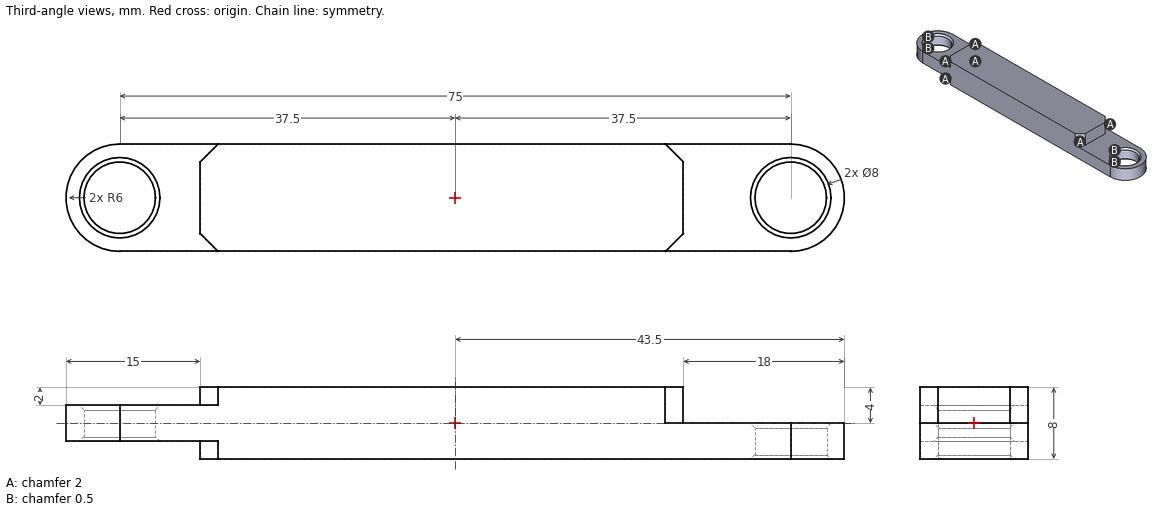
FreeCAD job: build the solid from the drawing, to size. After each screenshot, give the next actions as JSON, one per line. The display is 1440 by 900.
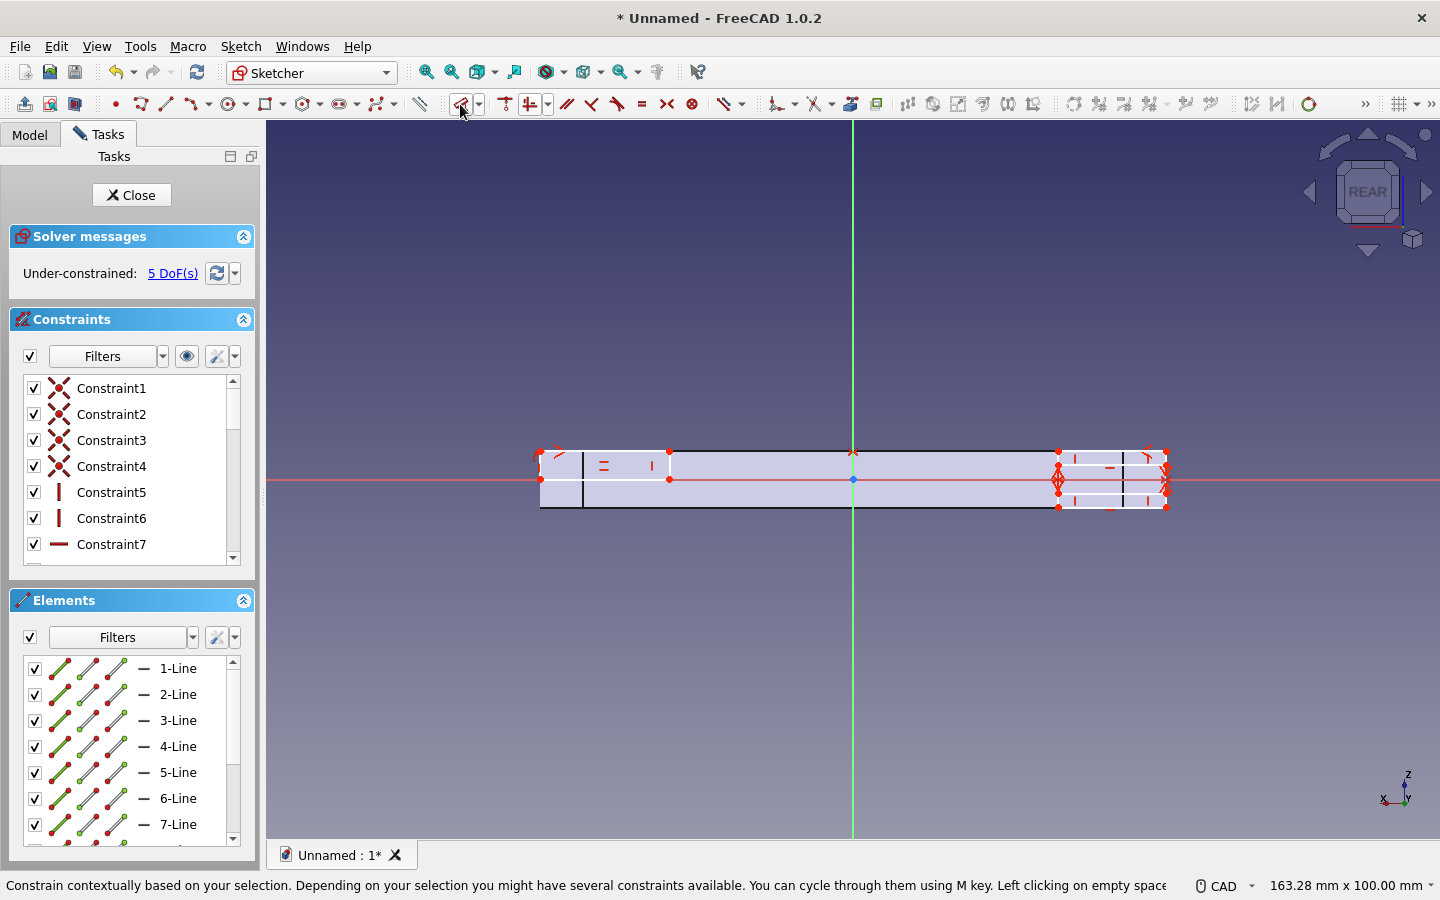
{"action": "scroll", "coordinate": [540, 463], "scroll_direction": "up", "scroll_amount": 2}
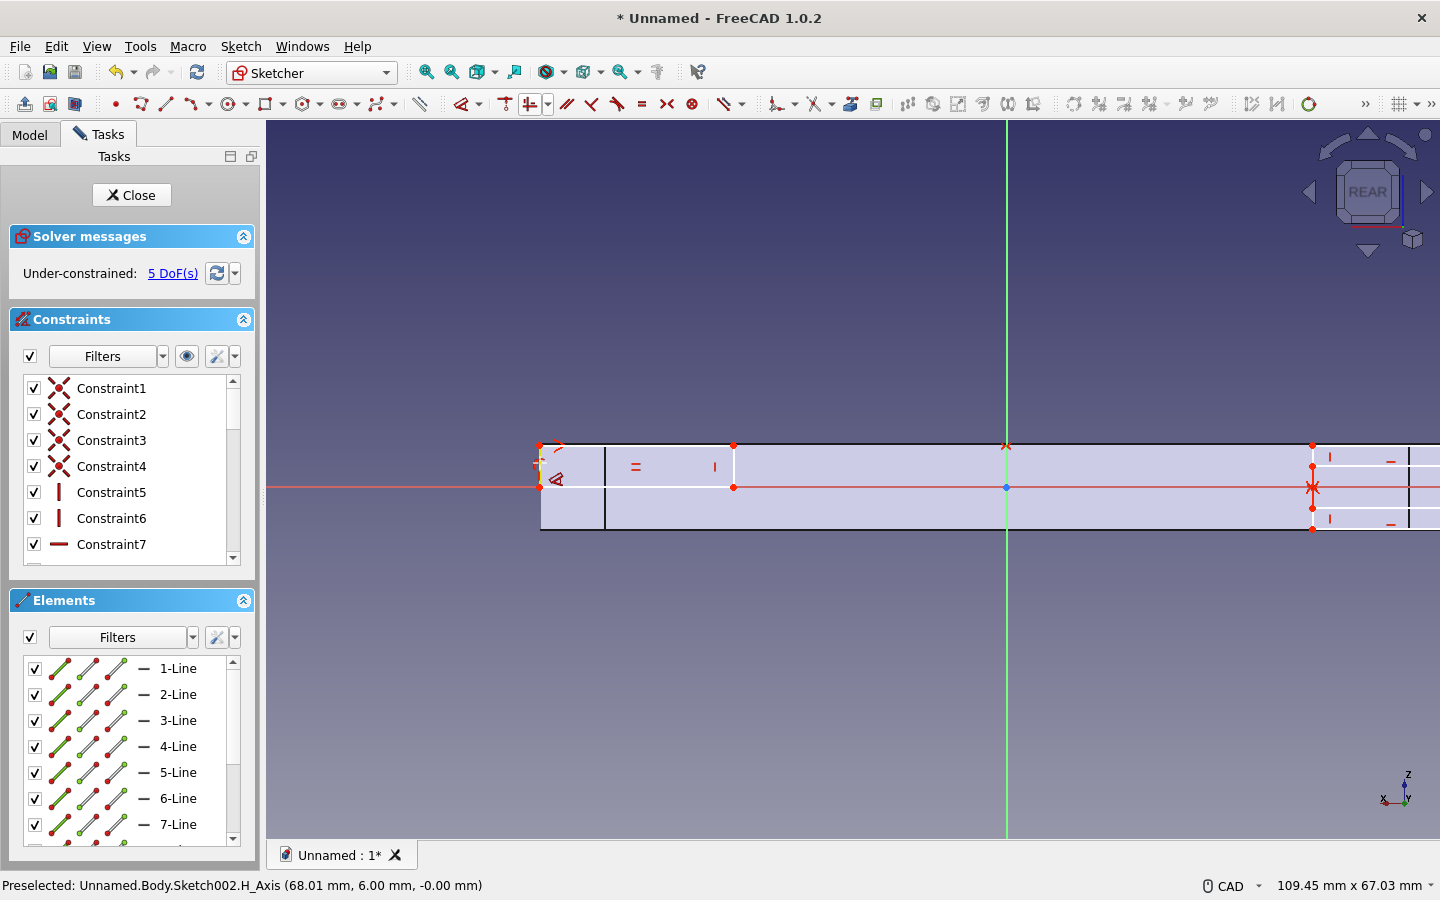
{"action": "left_click", "coordinate": [540, 462]}
{"action": "left_click", "coordinate": [506, 466]}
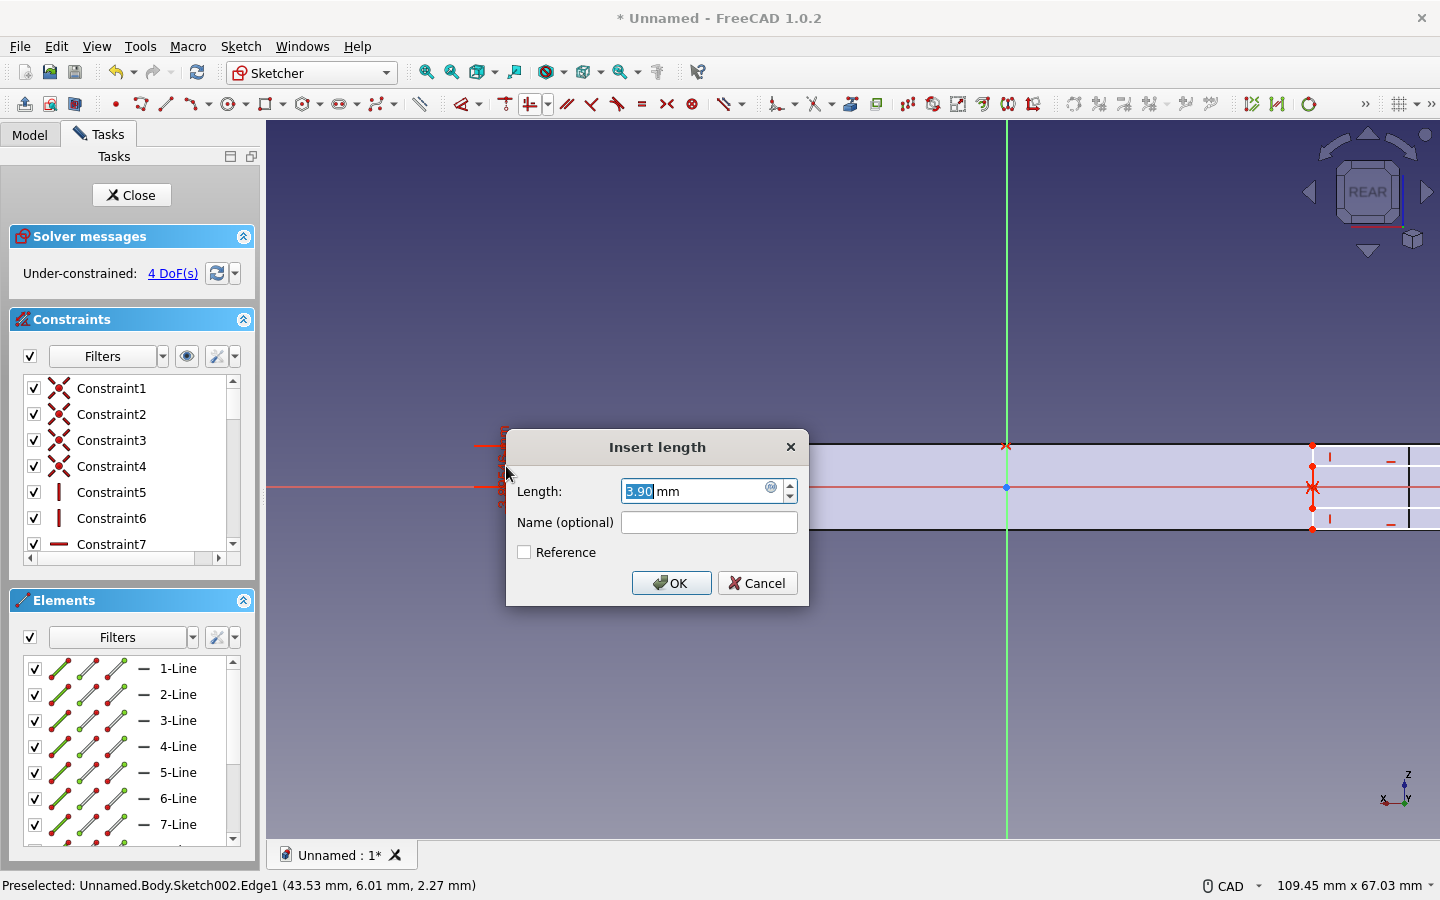
{"action": "type", "text": "4"}
{"action": "key", "text": "Return"}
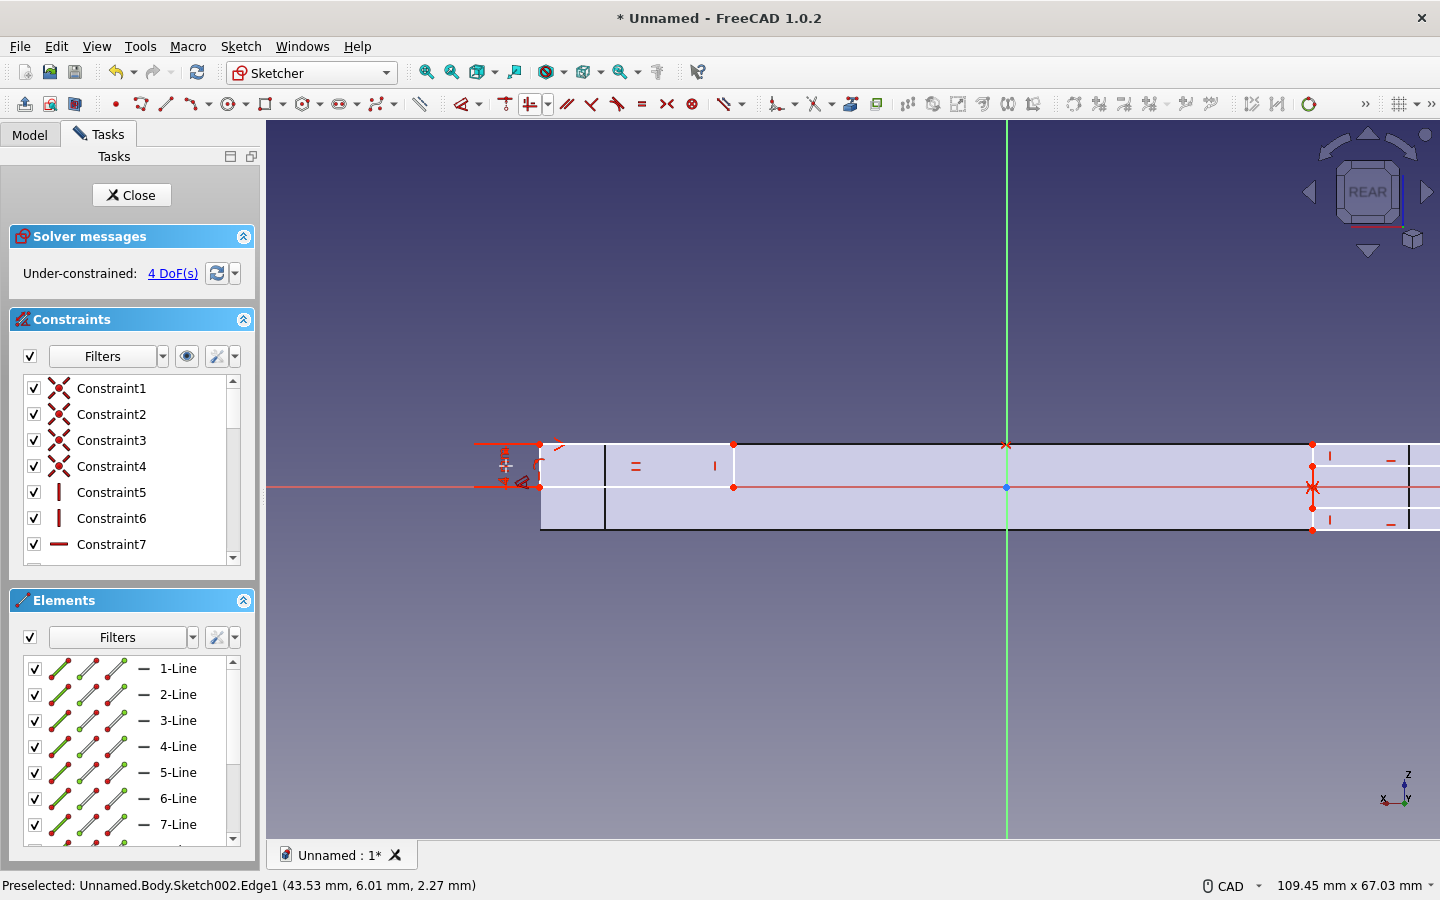
{"action": "scroll", "coordinate": [332, 463], "scroll_direction": "down", "scroll_amount": 2}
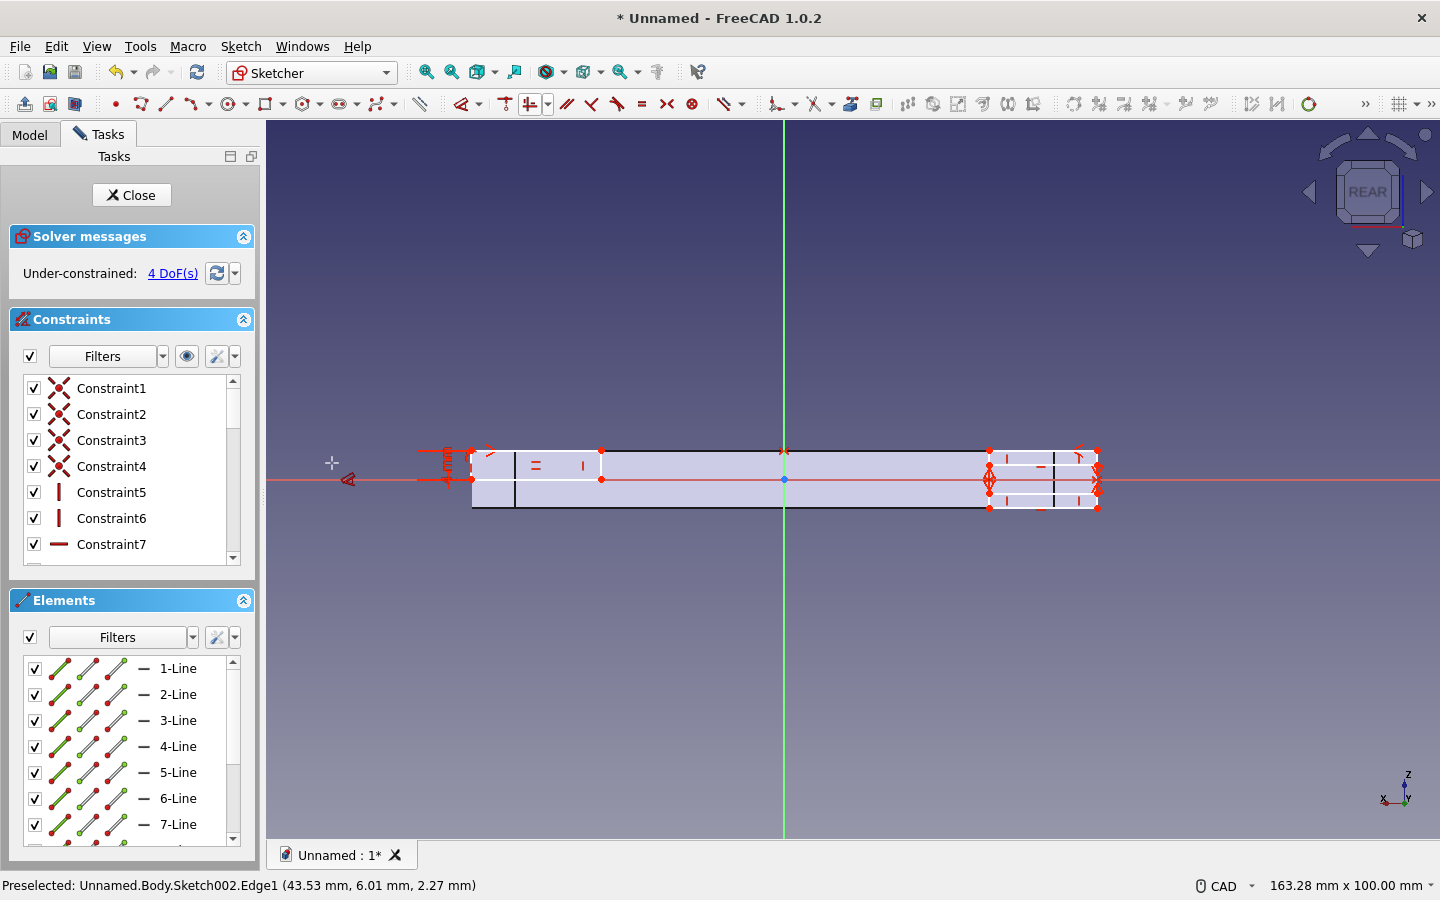
{"action": "scroll", "coordinate": [989, 458], "scroll_direction": "up", "scroll_amount": 6}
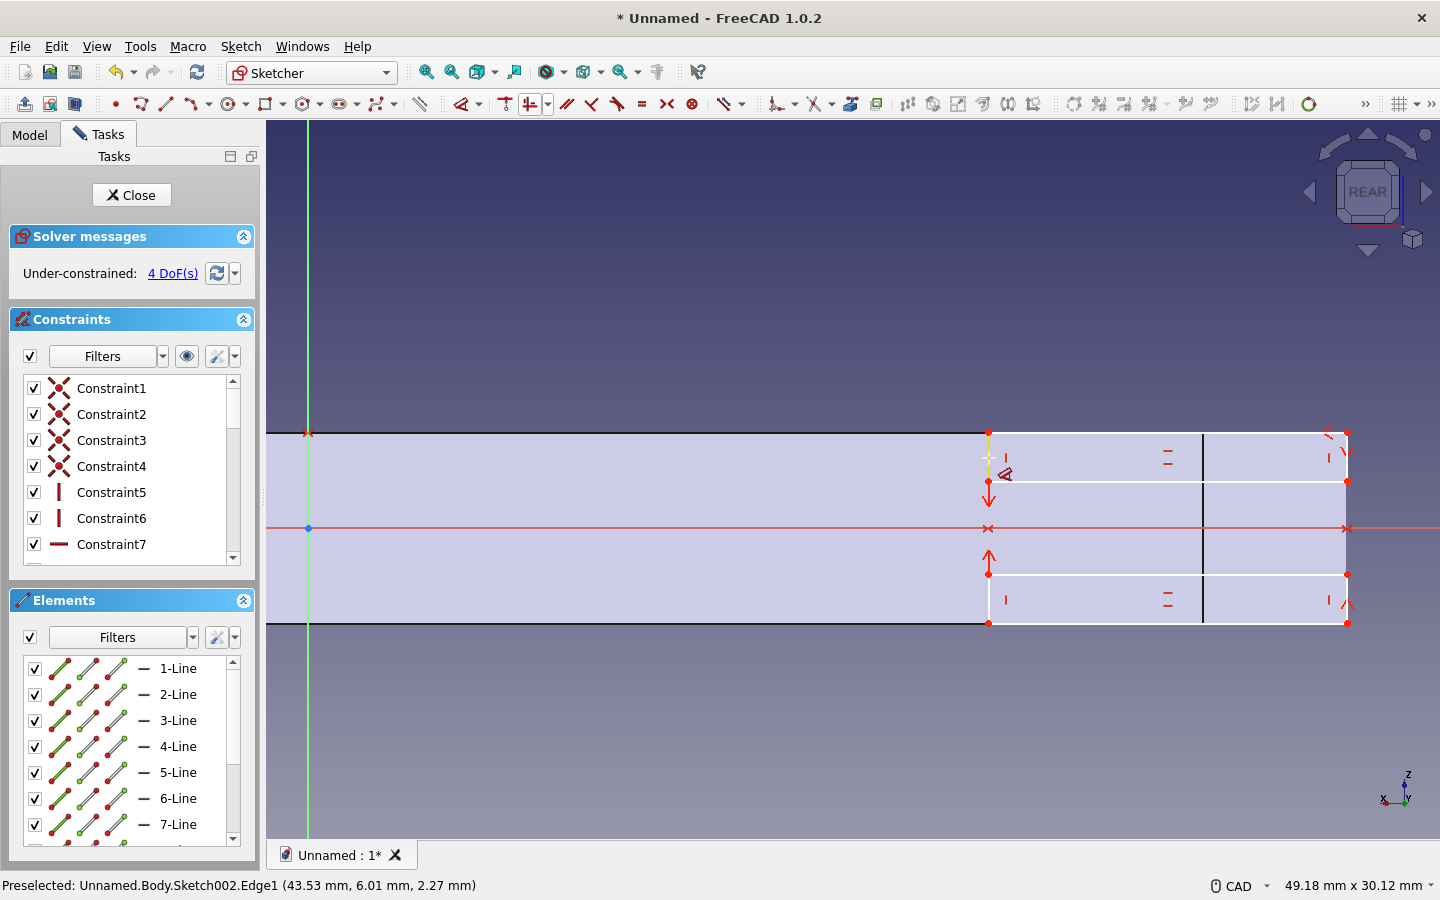
{"action": "left_click", "coordinate": [989, 457]}
{"action": "left_click", "coordinate": [1023, 457]}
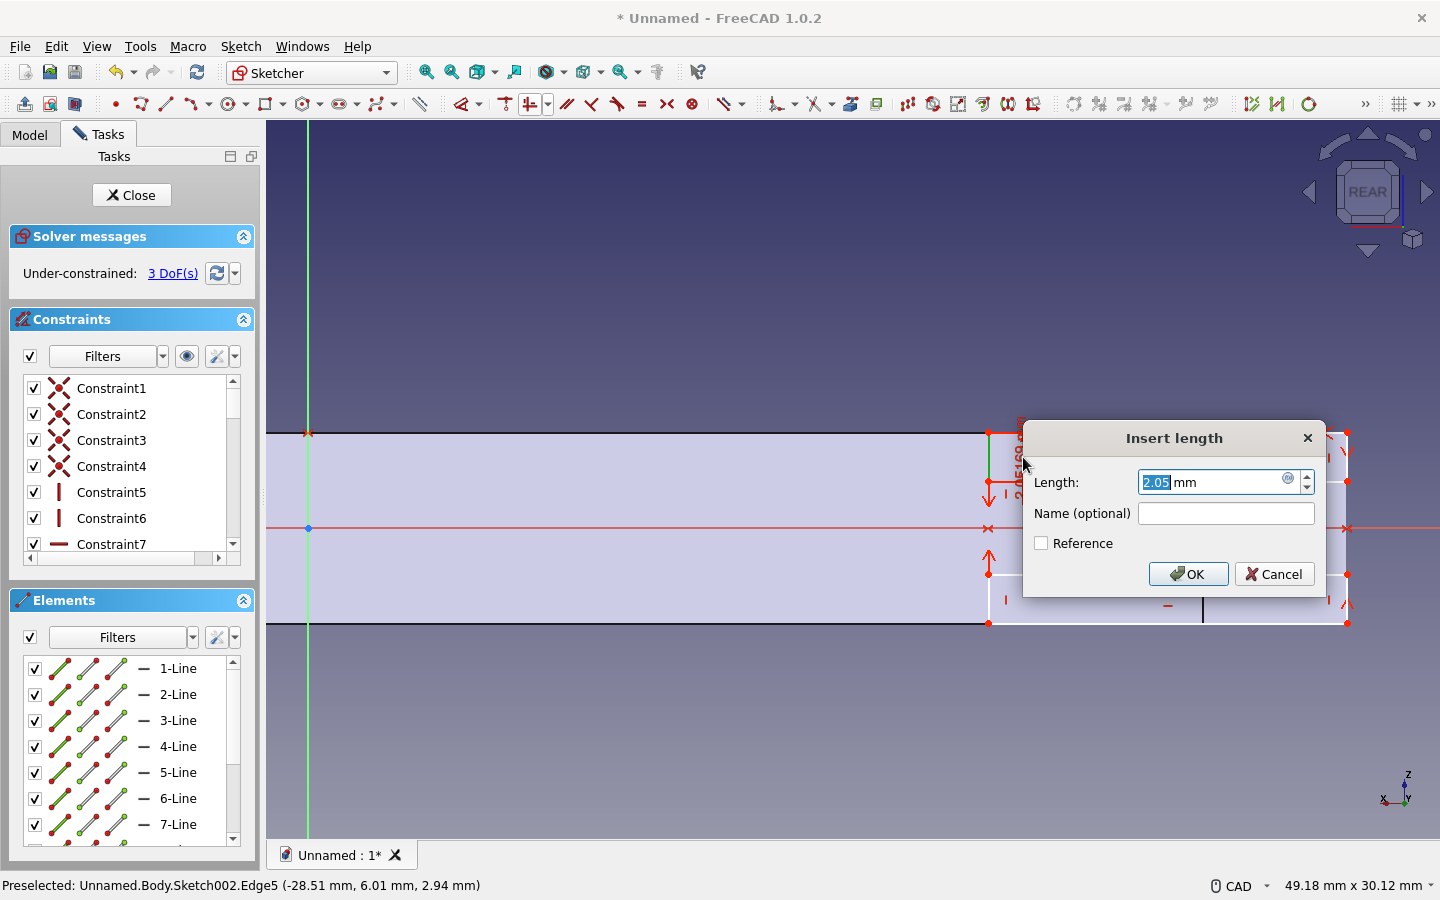
{"action": "type", "text": "2"}
{"action": "key", "text": "Return"}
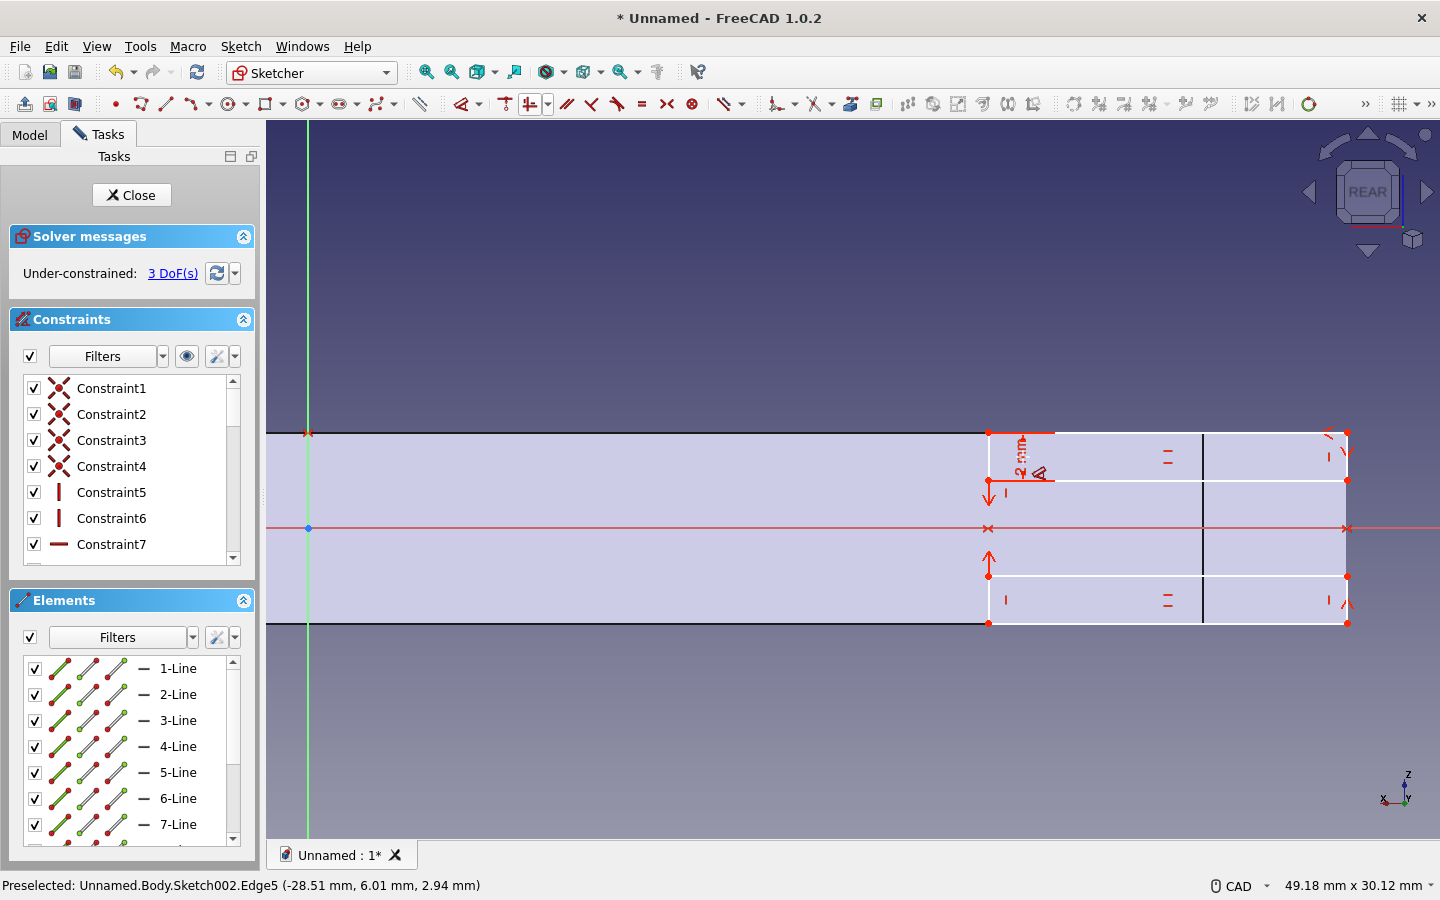
{"action": "scroll", "coordinate": [1062, 451], "scroll_direction": "down", "scroll_amount": 5}